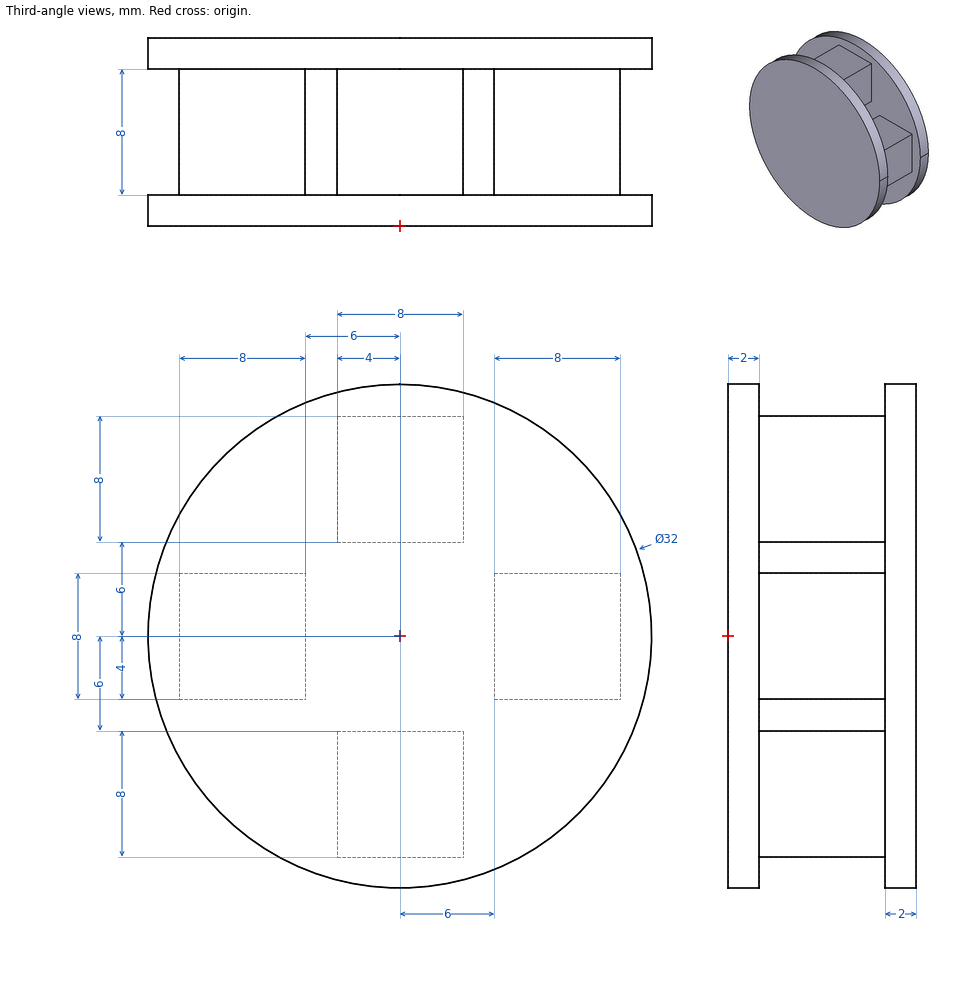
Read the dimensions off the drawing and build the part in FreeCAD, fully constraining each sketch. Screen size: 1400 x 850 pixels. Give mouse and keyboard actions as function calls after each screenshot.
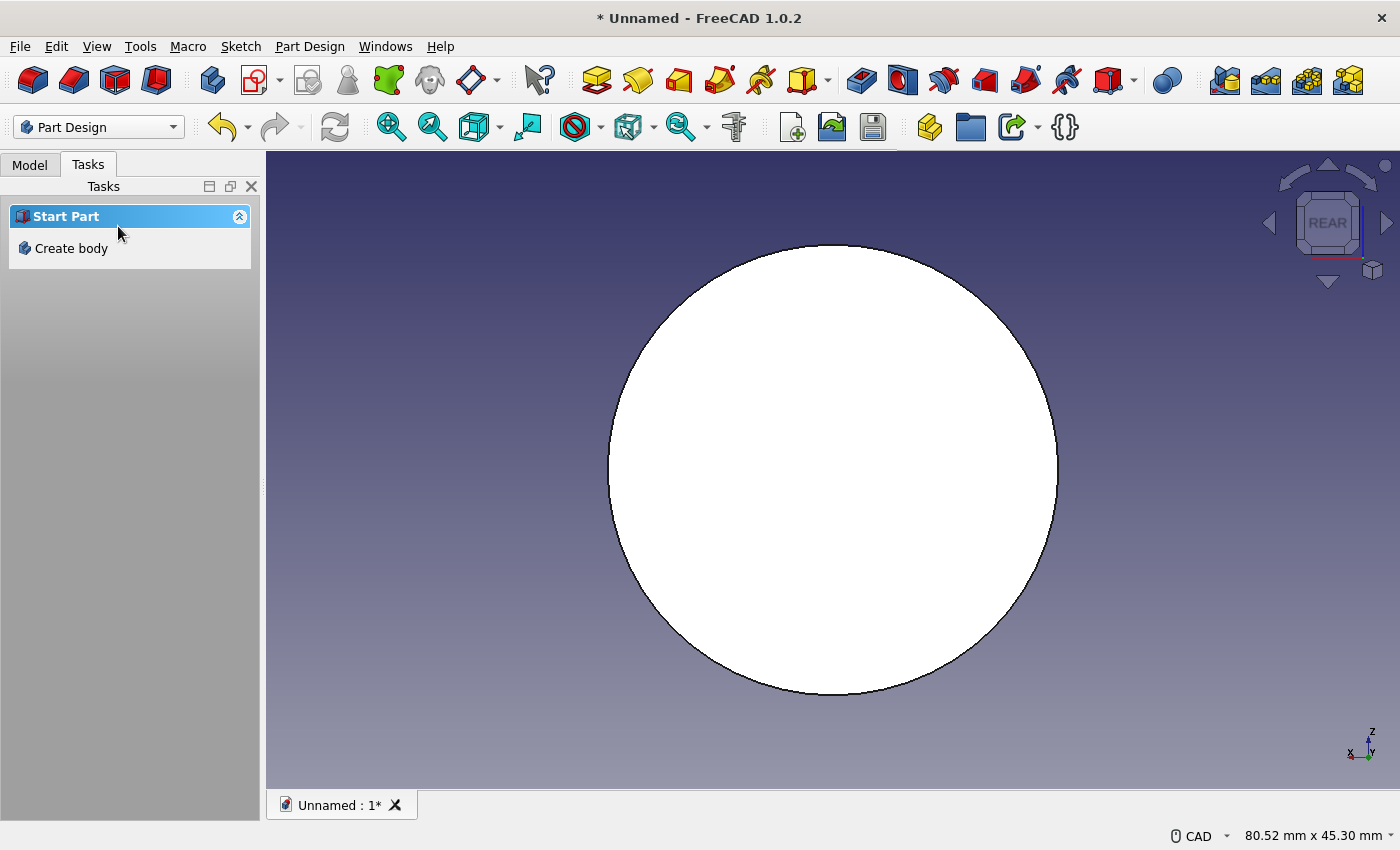
key(0)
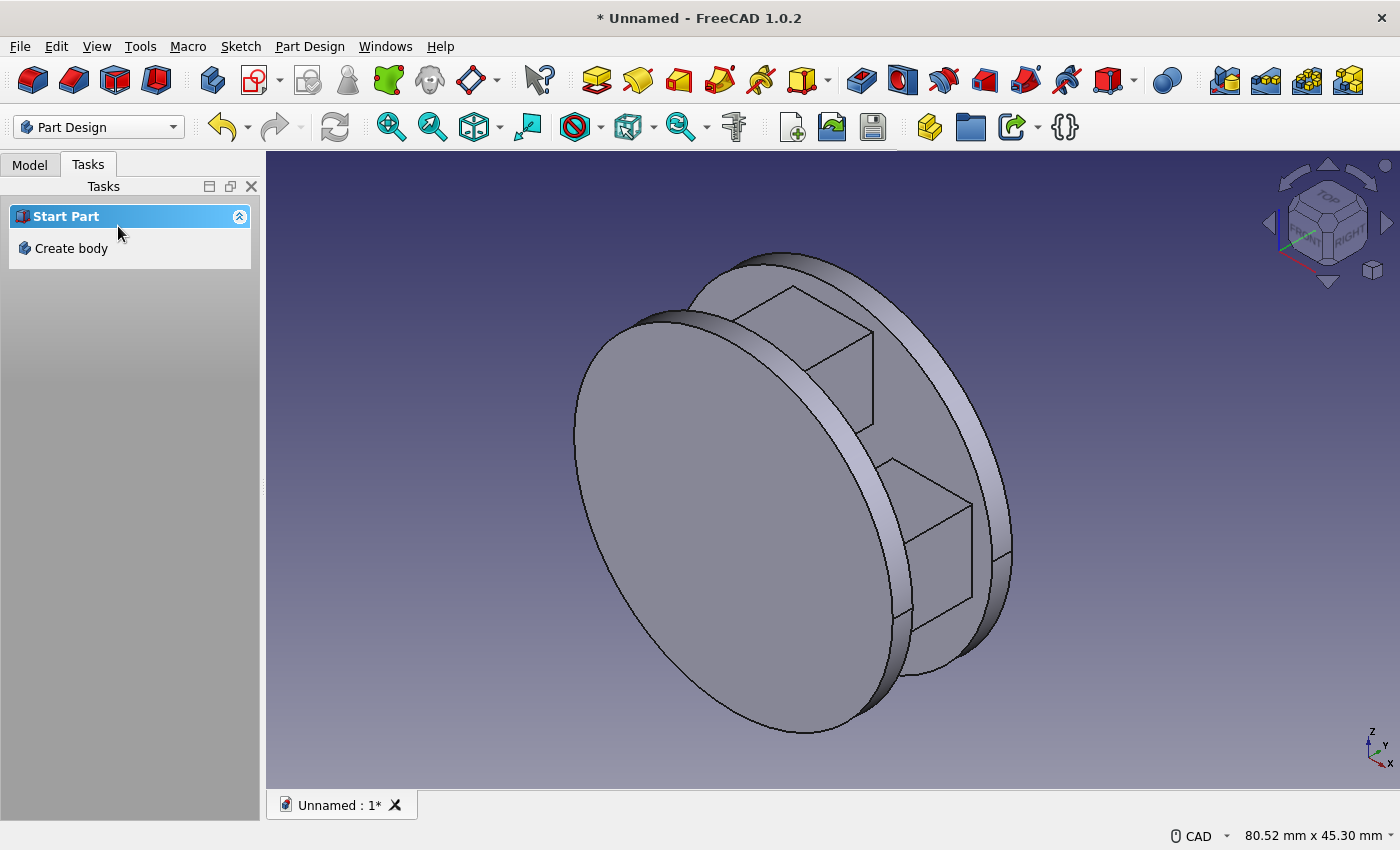
click(392, 128)